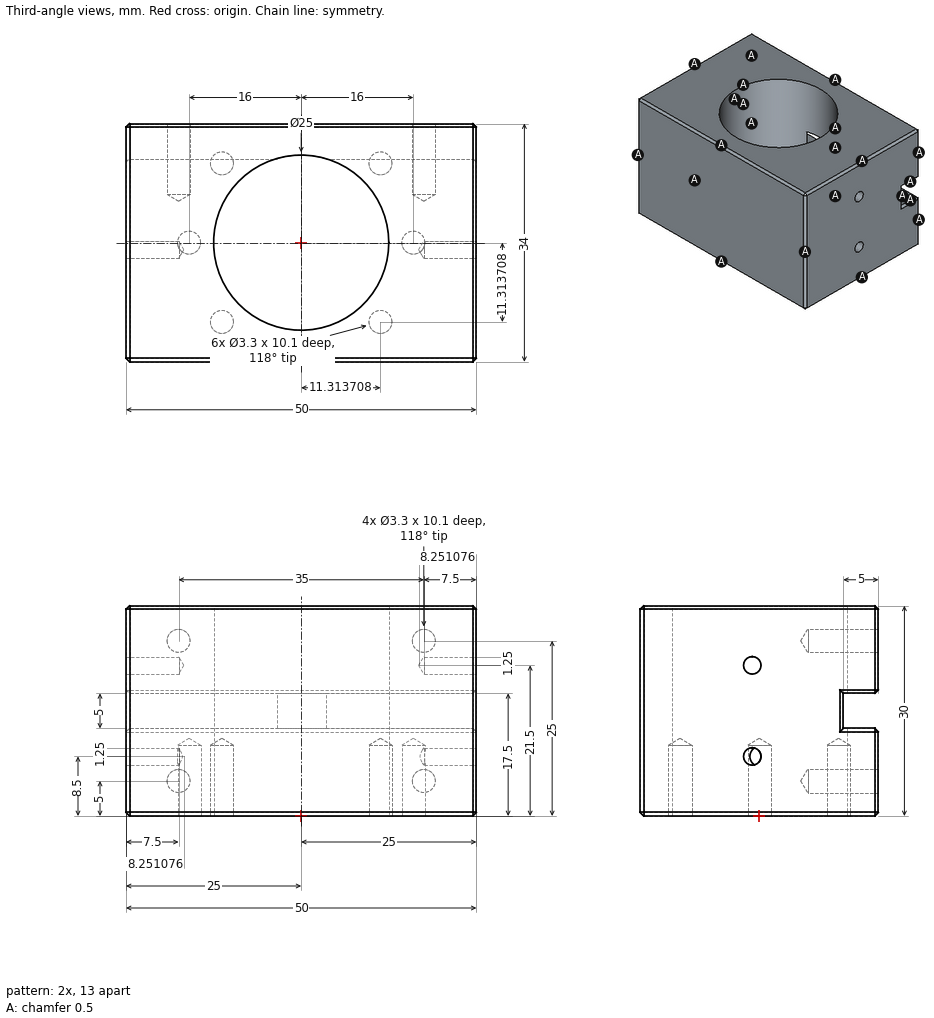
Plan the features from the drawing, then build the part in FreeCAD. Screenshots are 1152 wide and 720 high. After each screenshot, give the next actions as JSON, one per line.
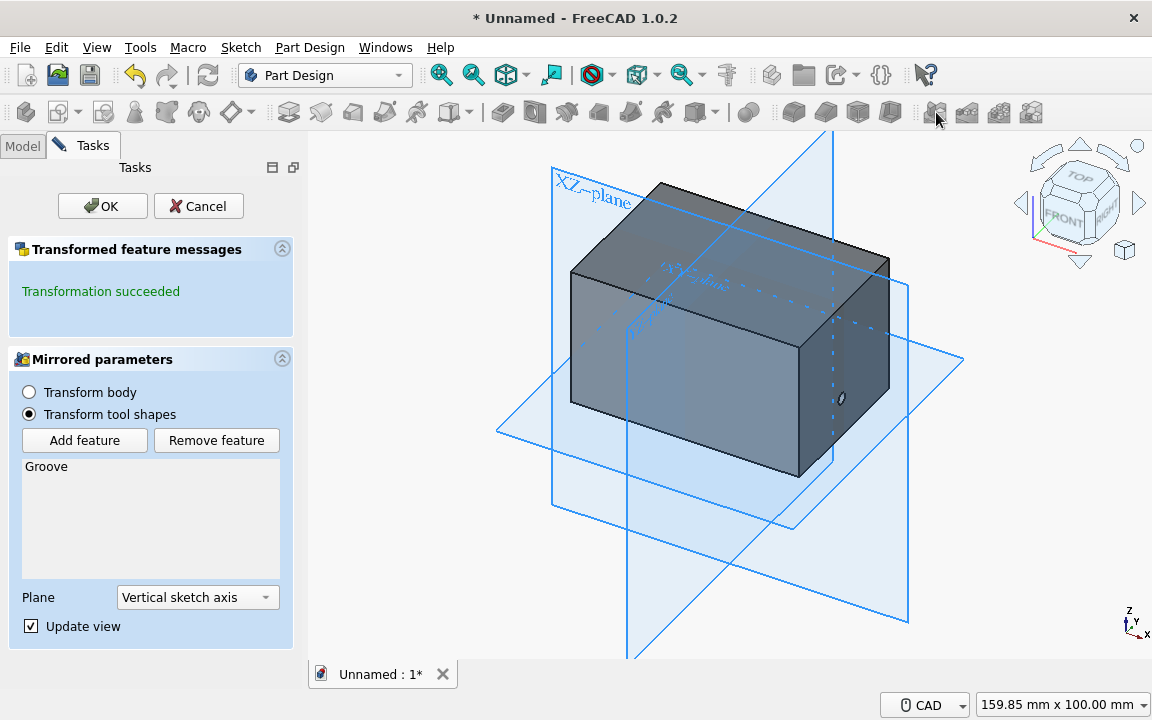
{"action": "left_click", "coordinate": [198, 598]}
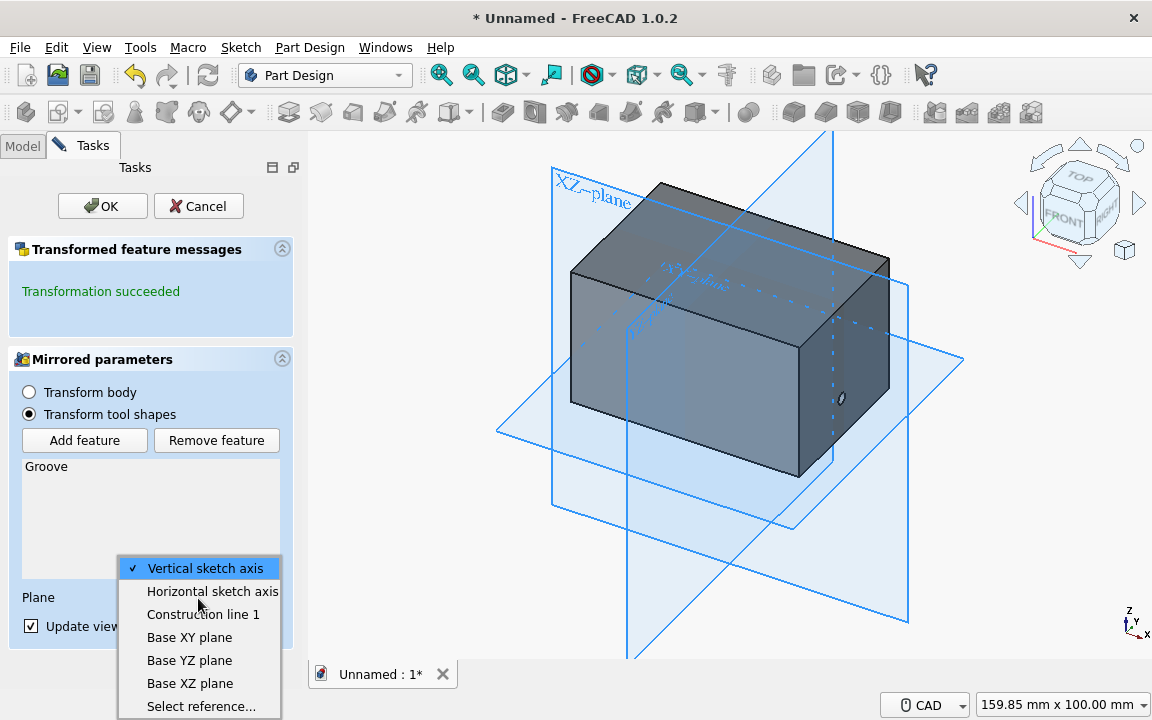
{"action": "left_click", "coordinate": [198, 660]}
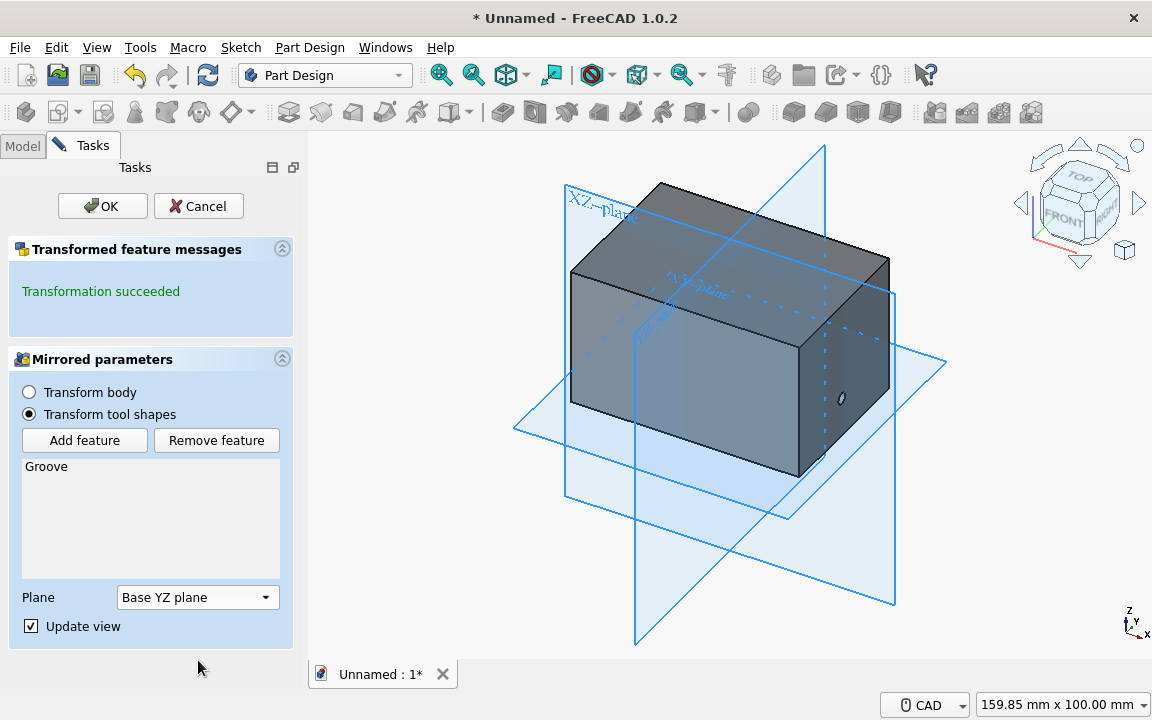
{"action": "left_click", "coordinate": [103, 206]}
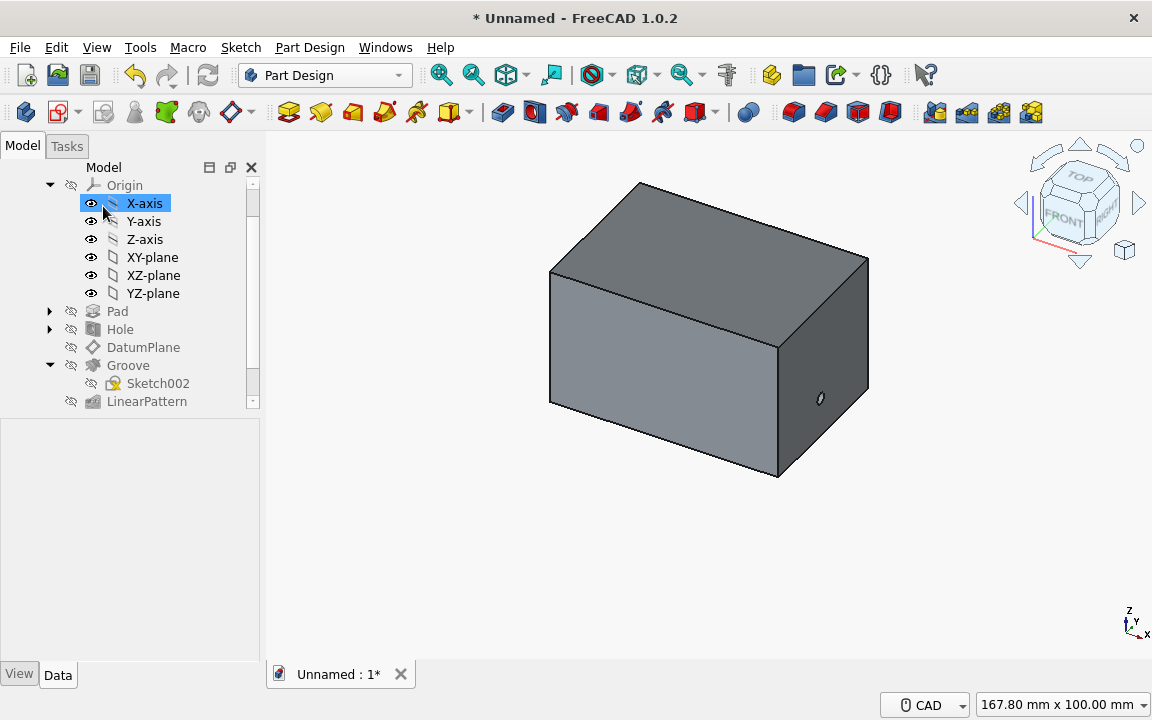
{"action": "left_click", "coordinate": [136, 275]}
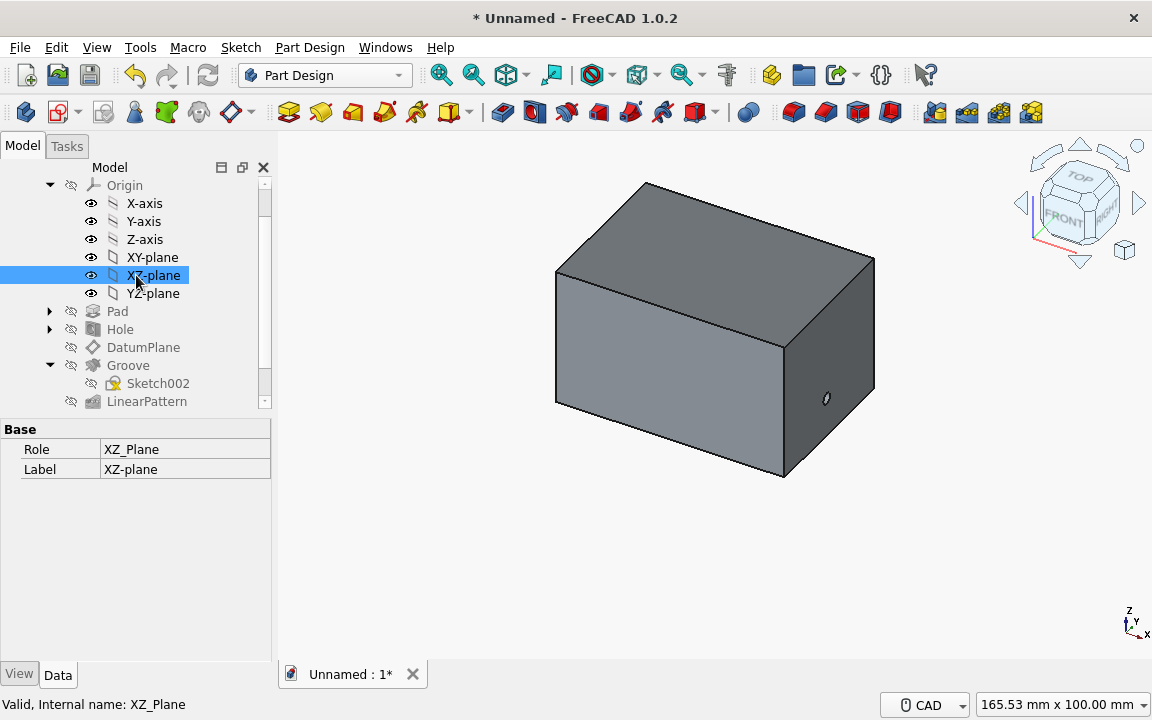
{"action": "left_click", "coordinate": [232, 112]}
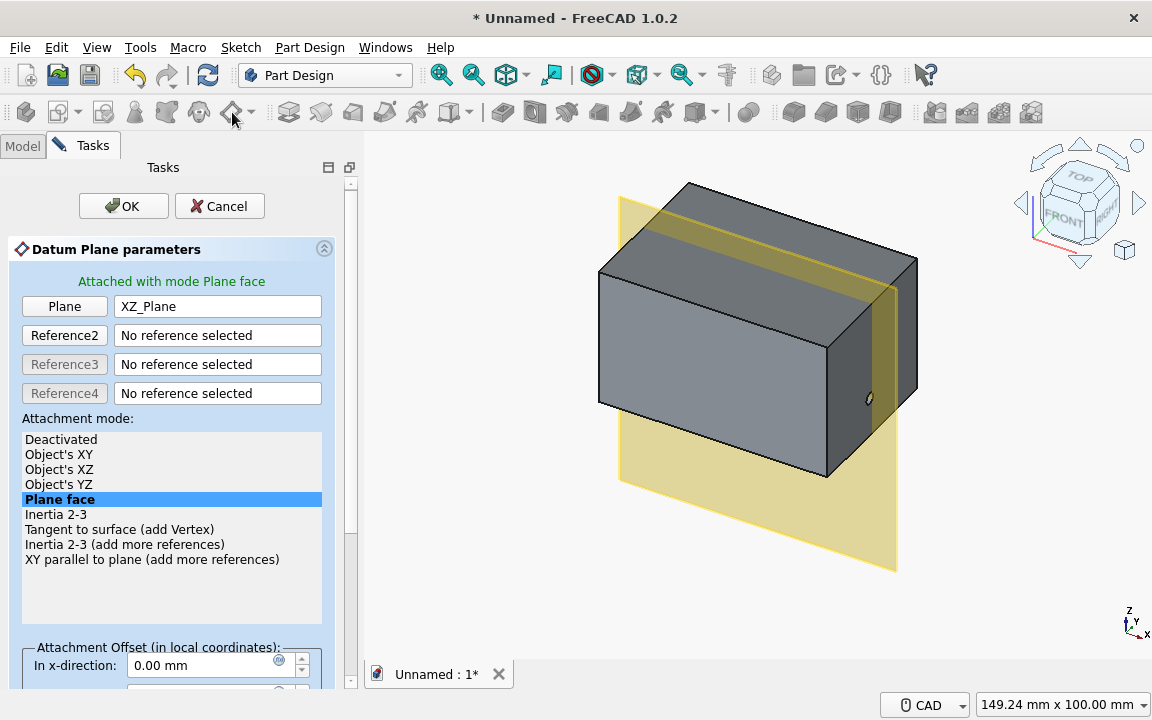
{"action": "scroll", "coordinate": [351, 432], "scroll_direction": "down", "scroll_amount": 2}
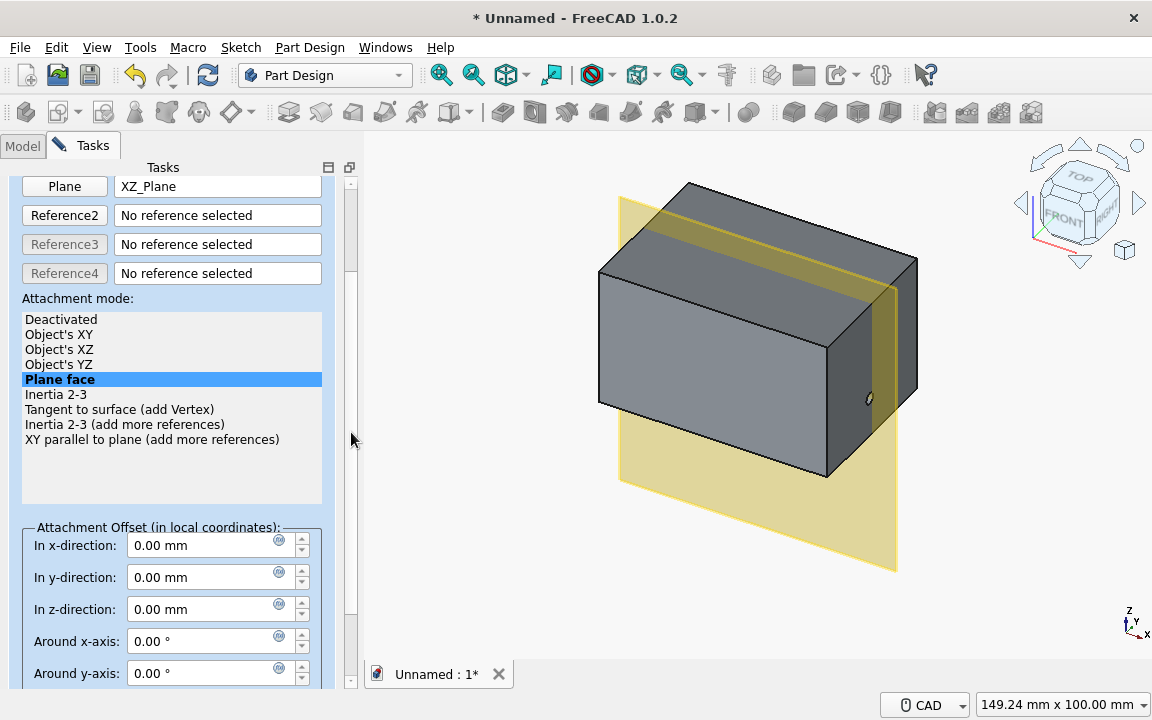
{"action": "triple_click", "coordinate": [210, 609]}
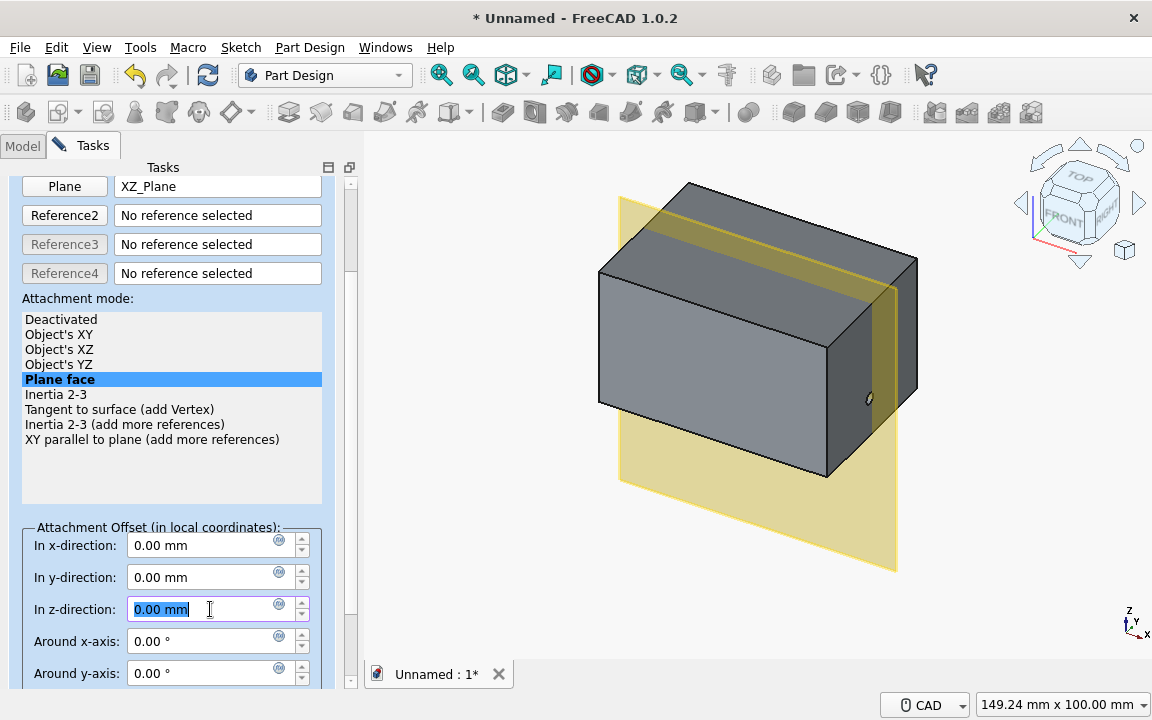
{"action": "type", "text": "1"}
{"action": "key", "text": "Tab"}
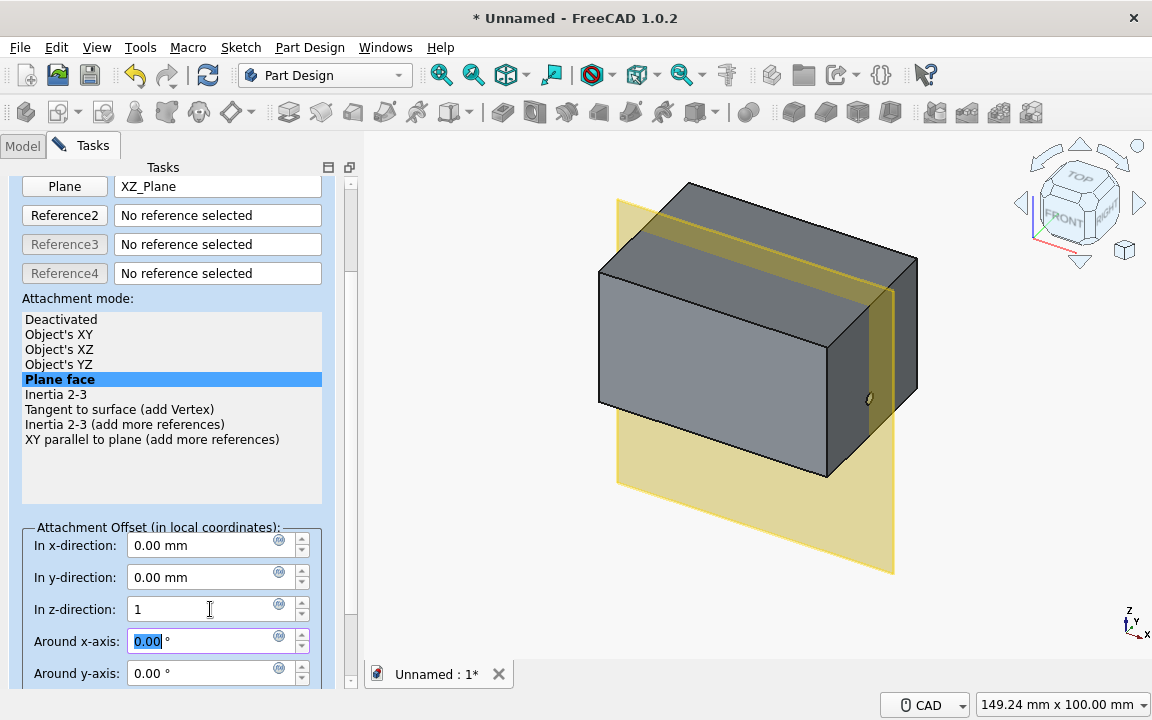
{"action": "scroll", "coordinate": [351, 432], "scroll_direction": "up", "scroll_amount": 3}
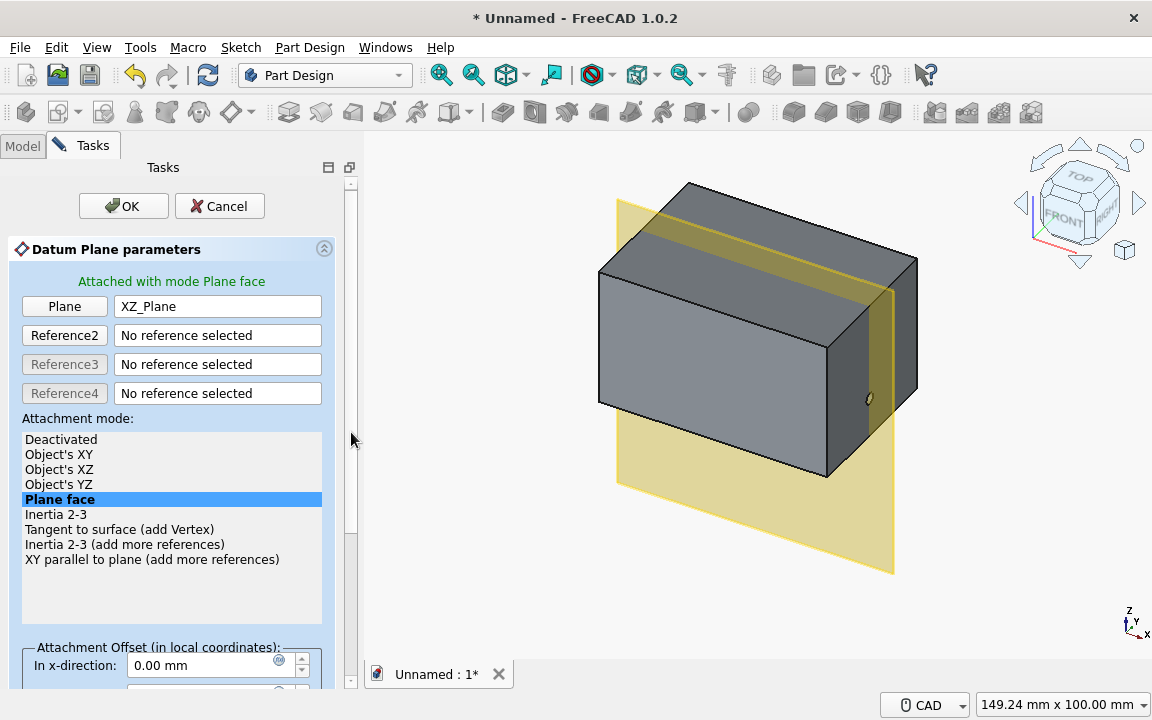
{"action": "left_click", "coordinate": [124, 206]}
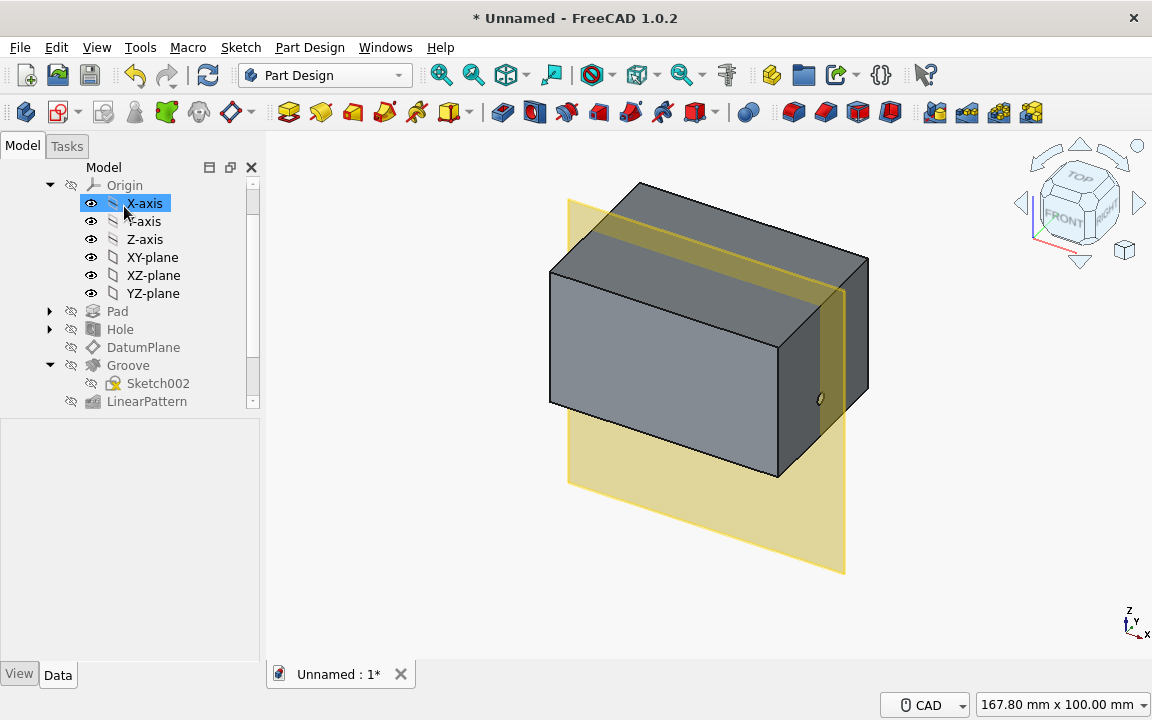
{"action": "scroll", "coordinate": [140, 289], "scroll_direction": "down", "scroll_amount": 3}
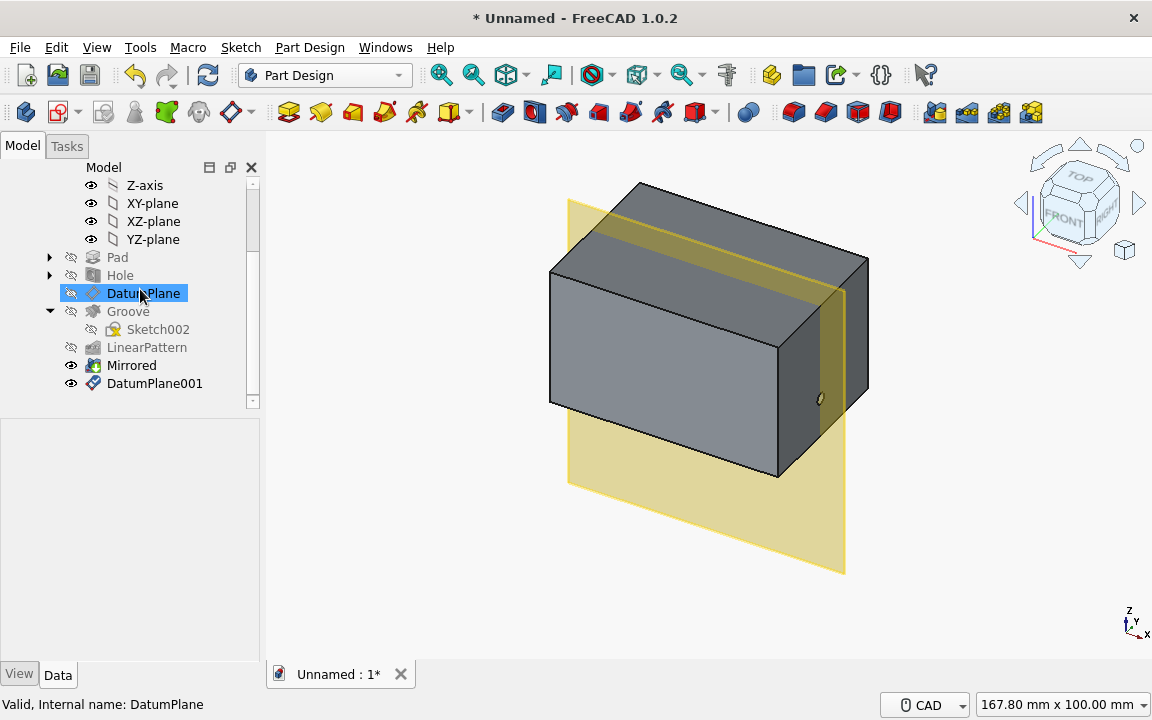
{"action": "left_click", "coordinate": [116, 383]}